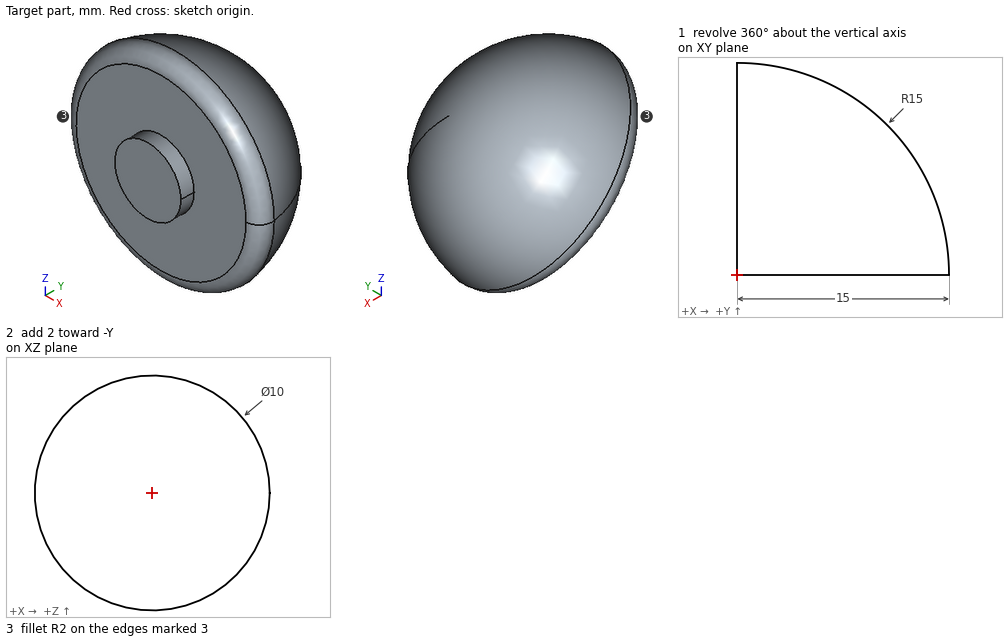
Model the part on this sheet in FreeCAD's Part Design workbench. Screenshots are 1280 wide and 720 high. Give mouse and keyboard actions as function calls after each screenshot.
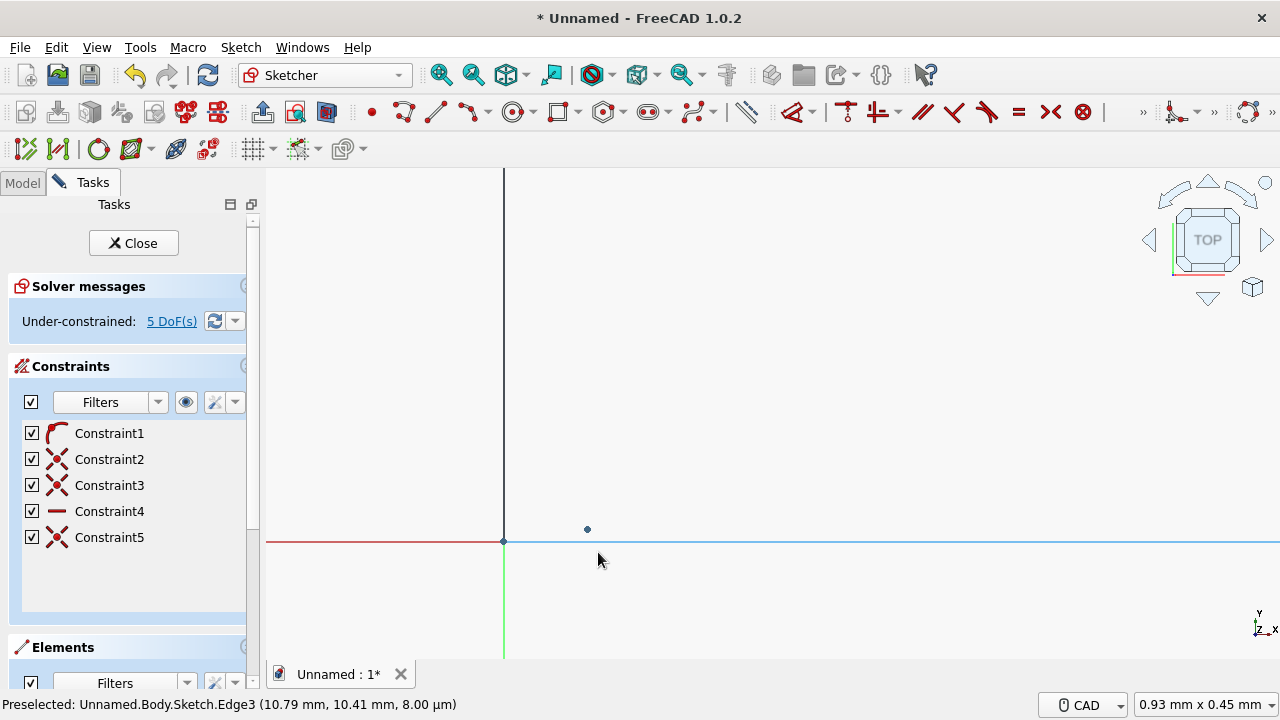
key(c)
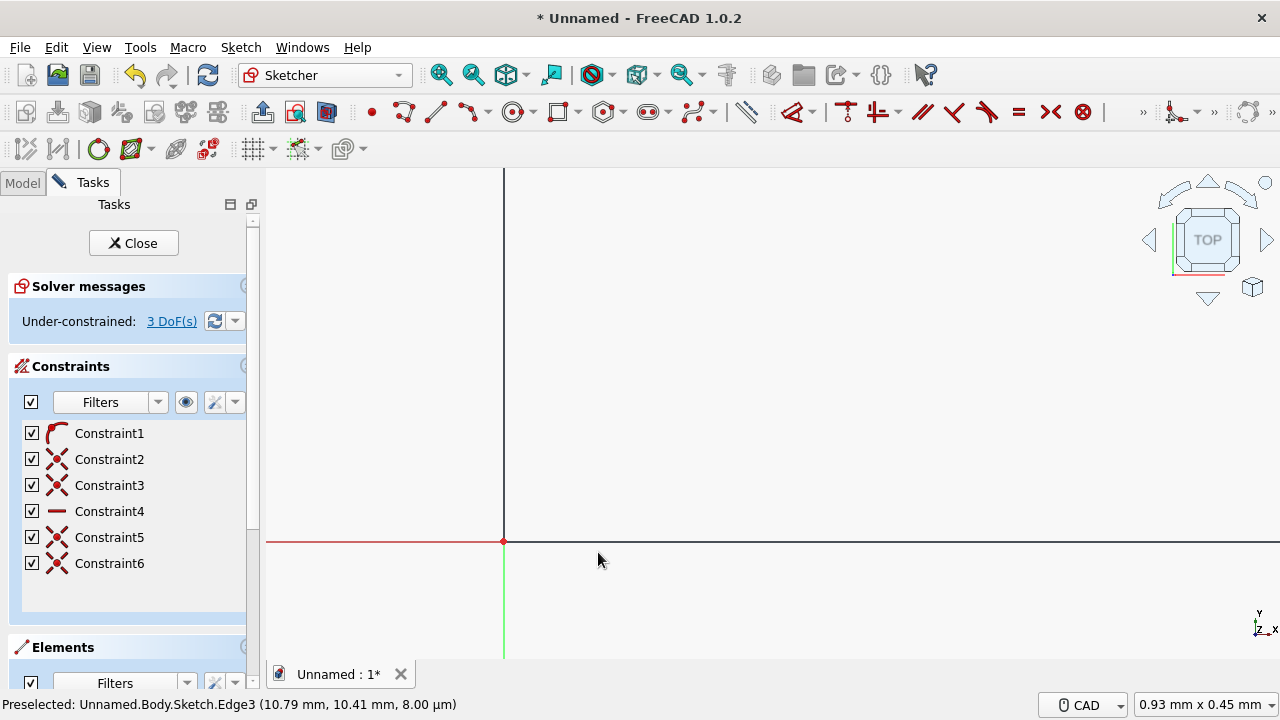
key(d)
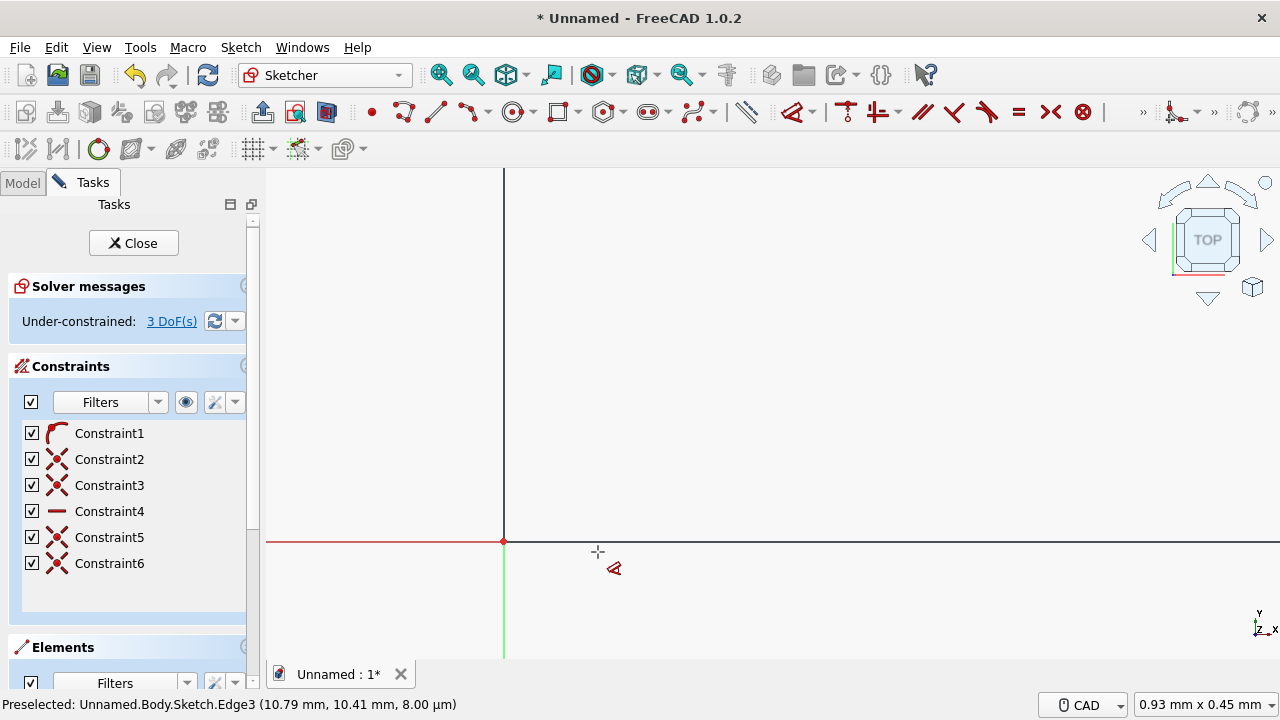
scroll(704, 414, down, 15)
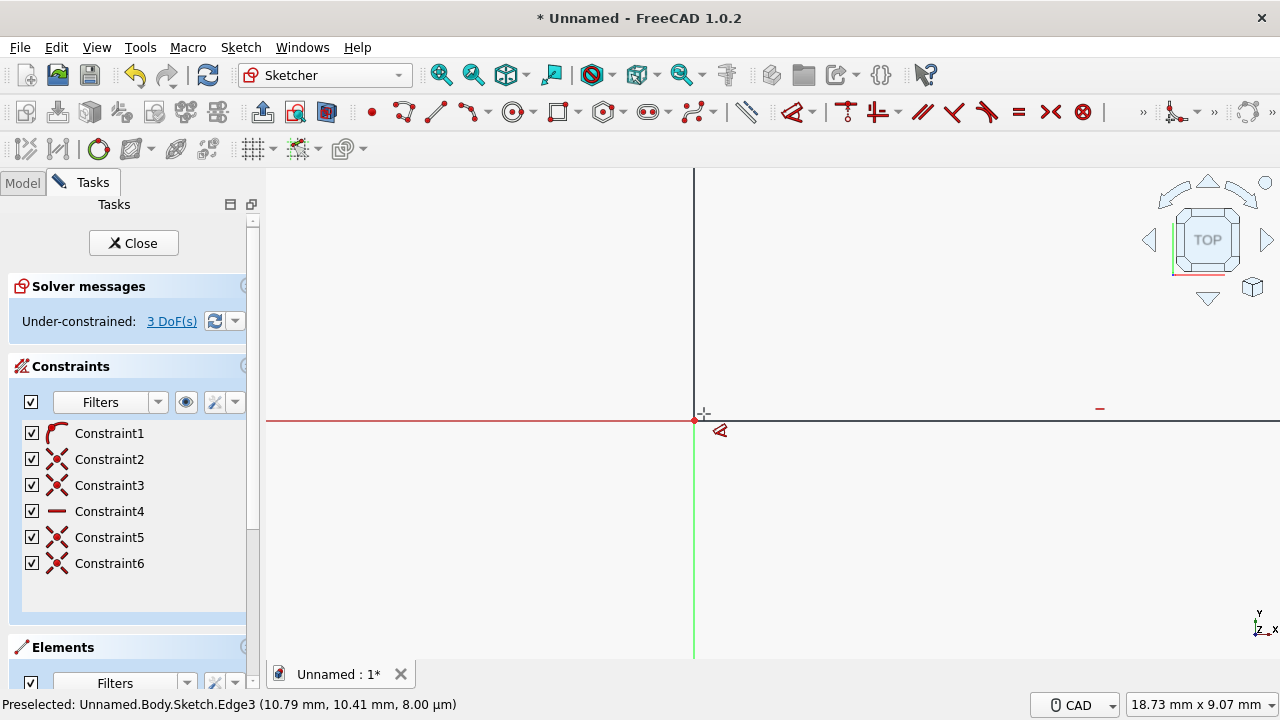
scroll(474, 631, down, 5)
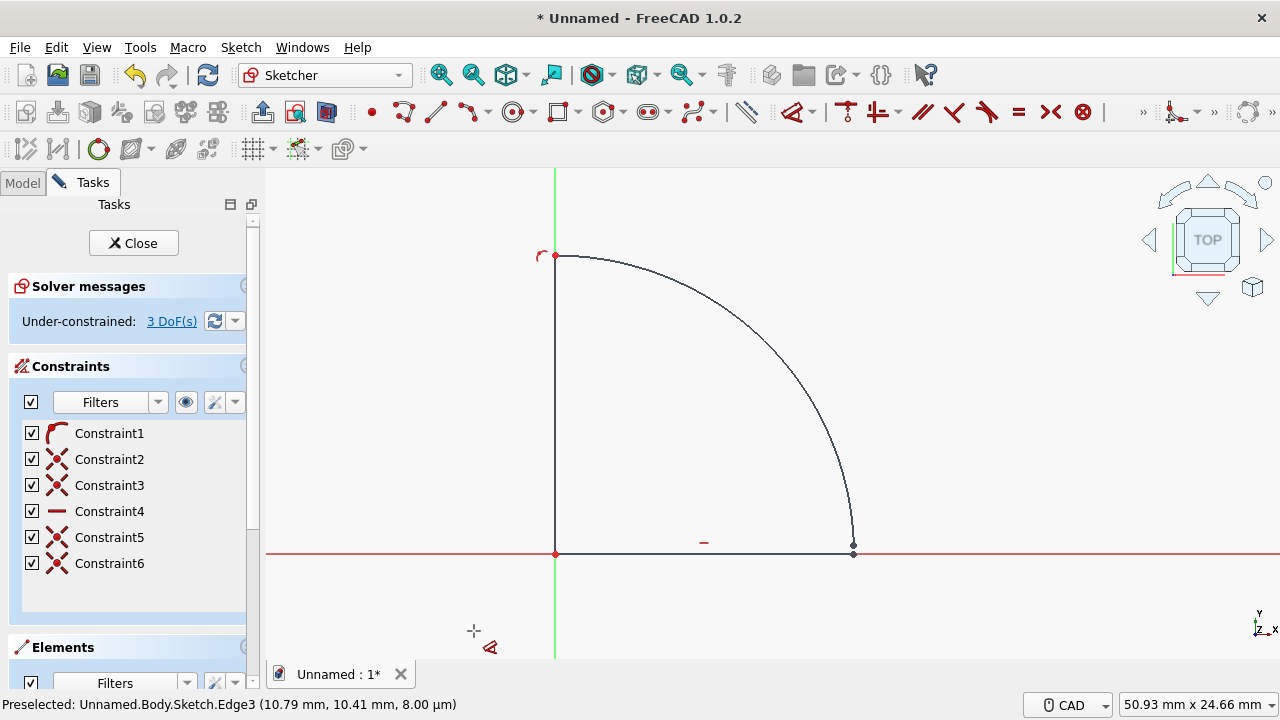
click(819, 413)
click(847, 398)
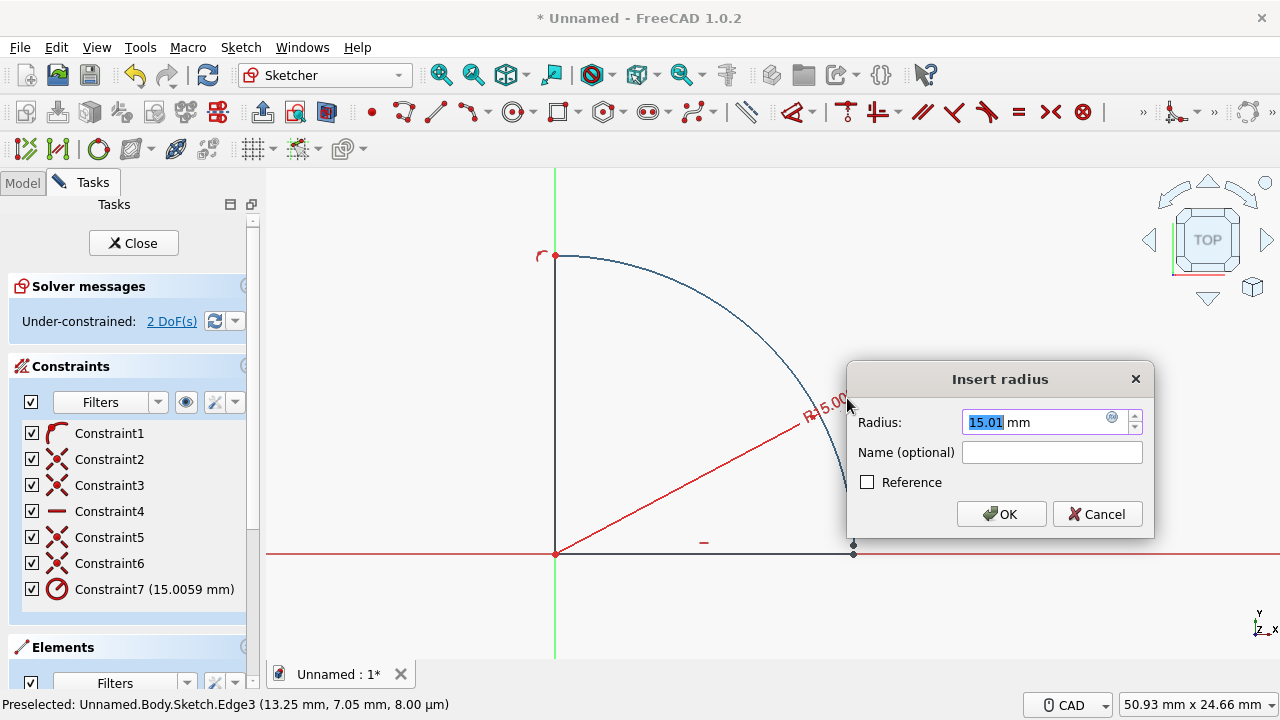
text(15)
key(Return)
key(Escape)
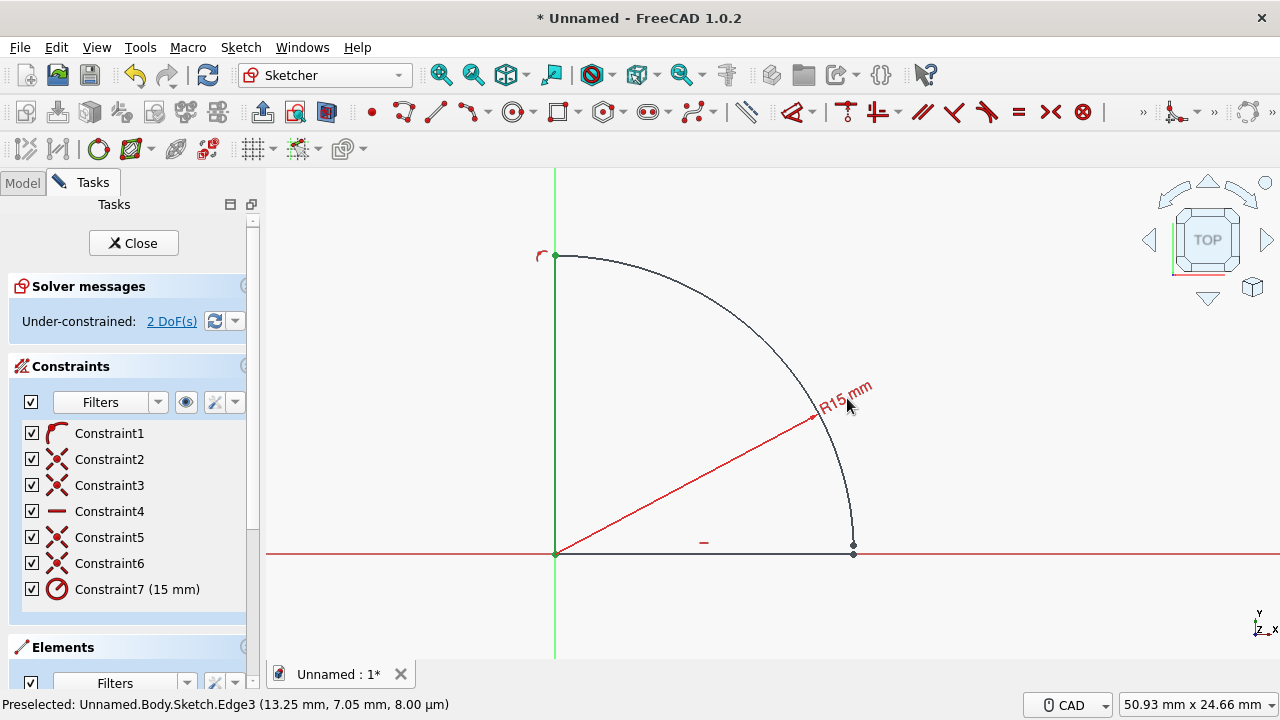
click(854, 546)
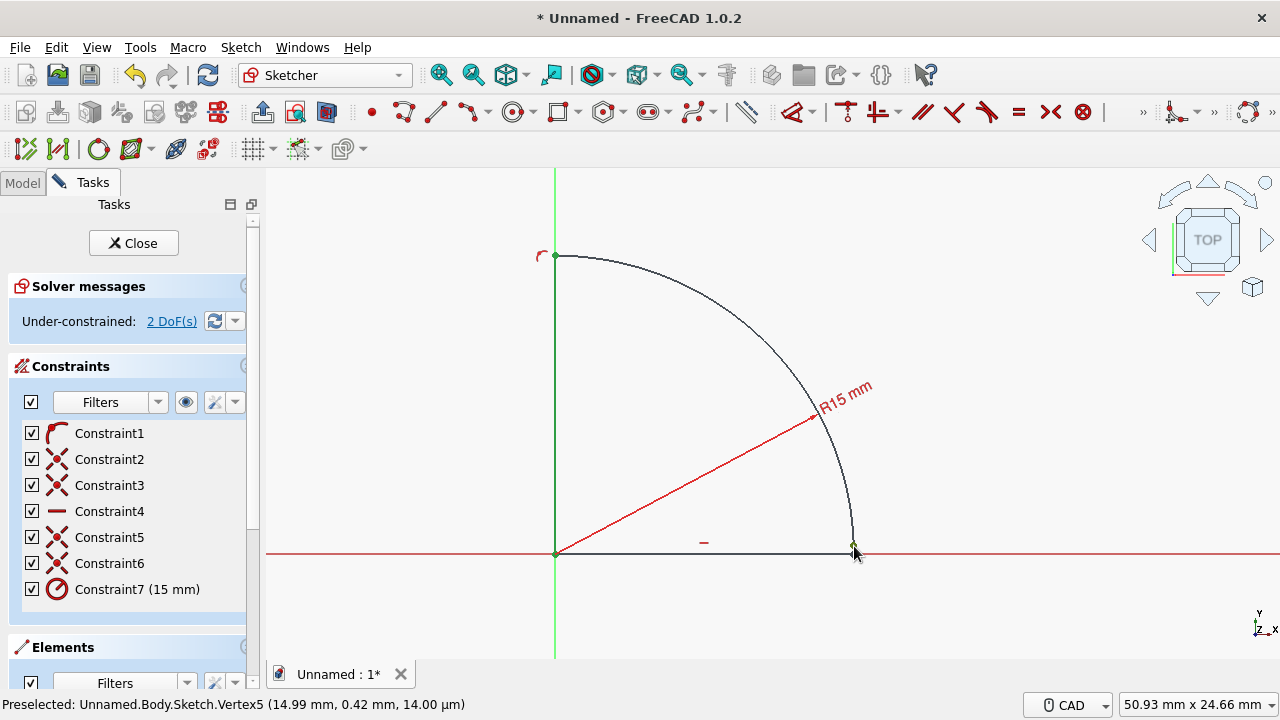
click(353, 554)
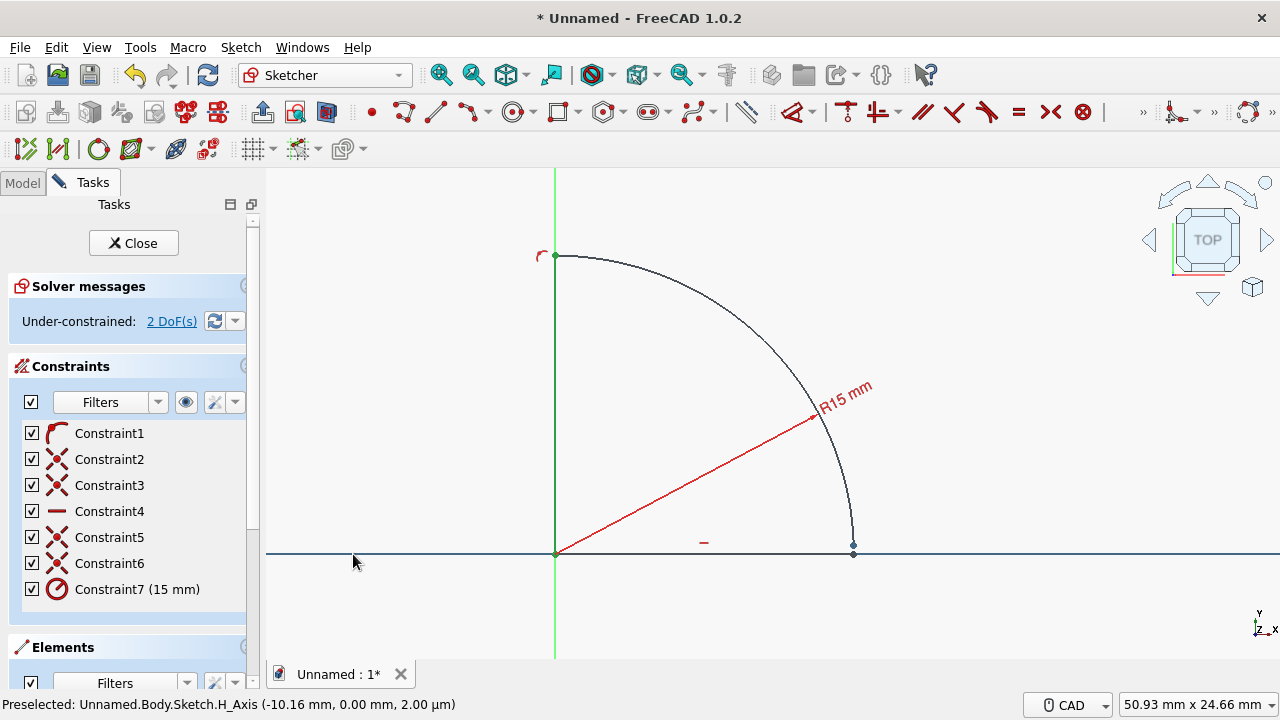
key(c)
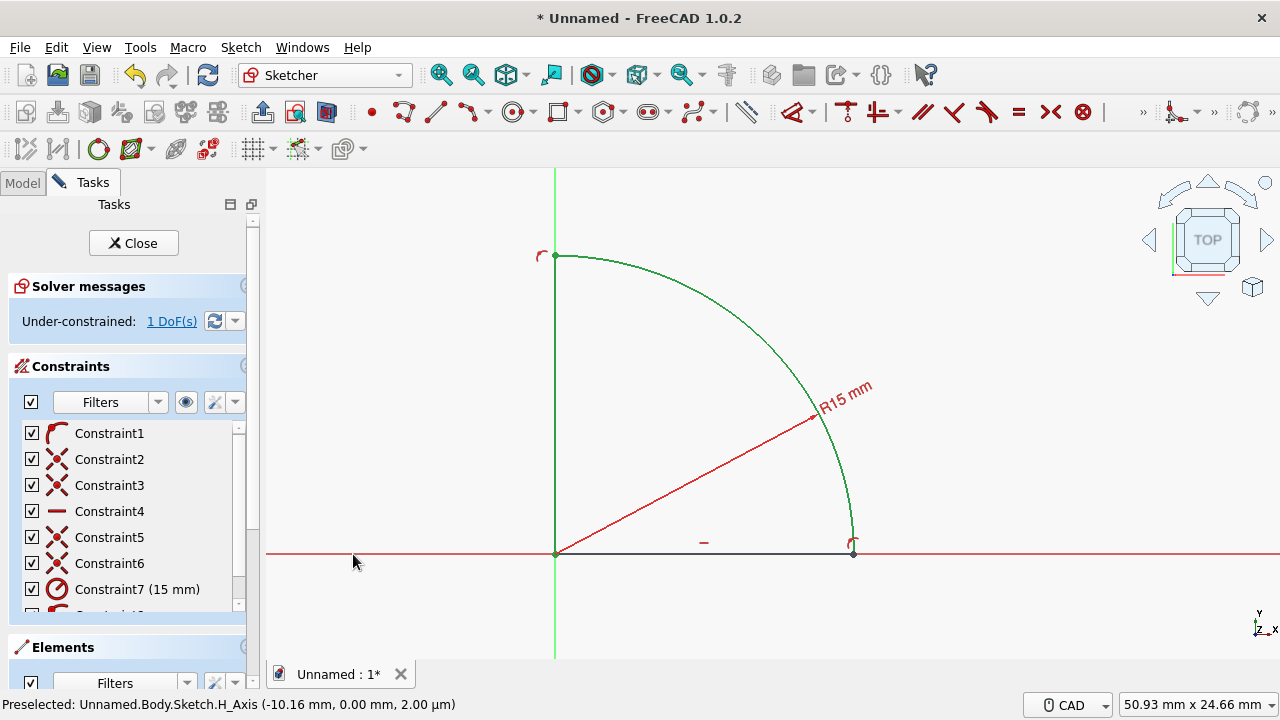
click(792, 112)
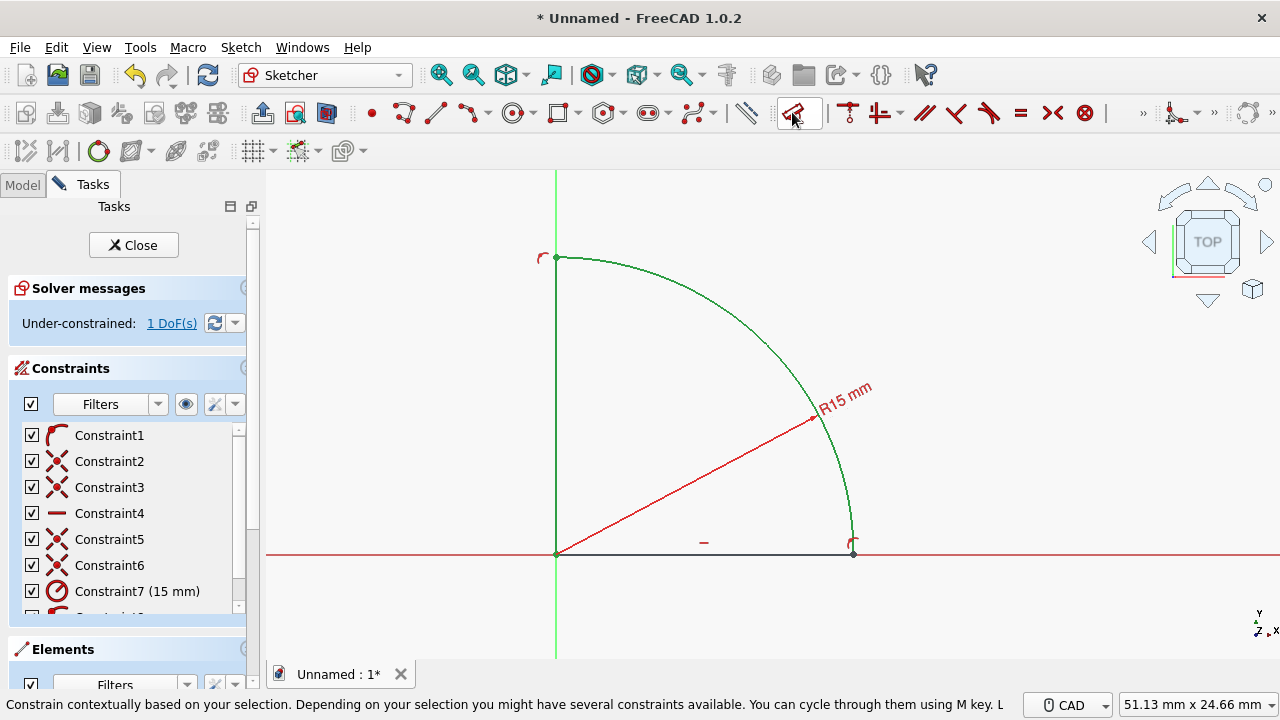
click(645, 555)
click(705, 589)